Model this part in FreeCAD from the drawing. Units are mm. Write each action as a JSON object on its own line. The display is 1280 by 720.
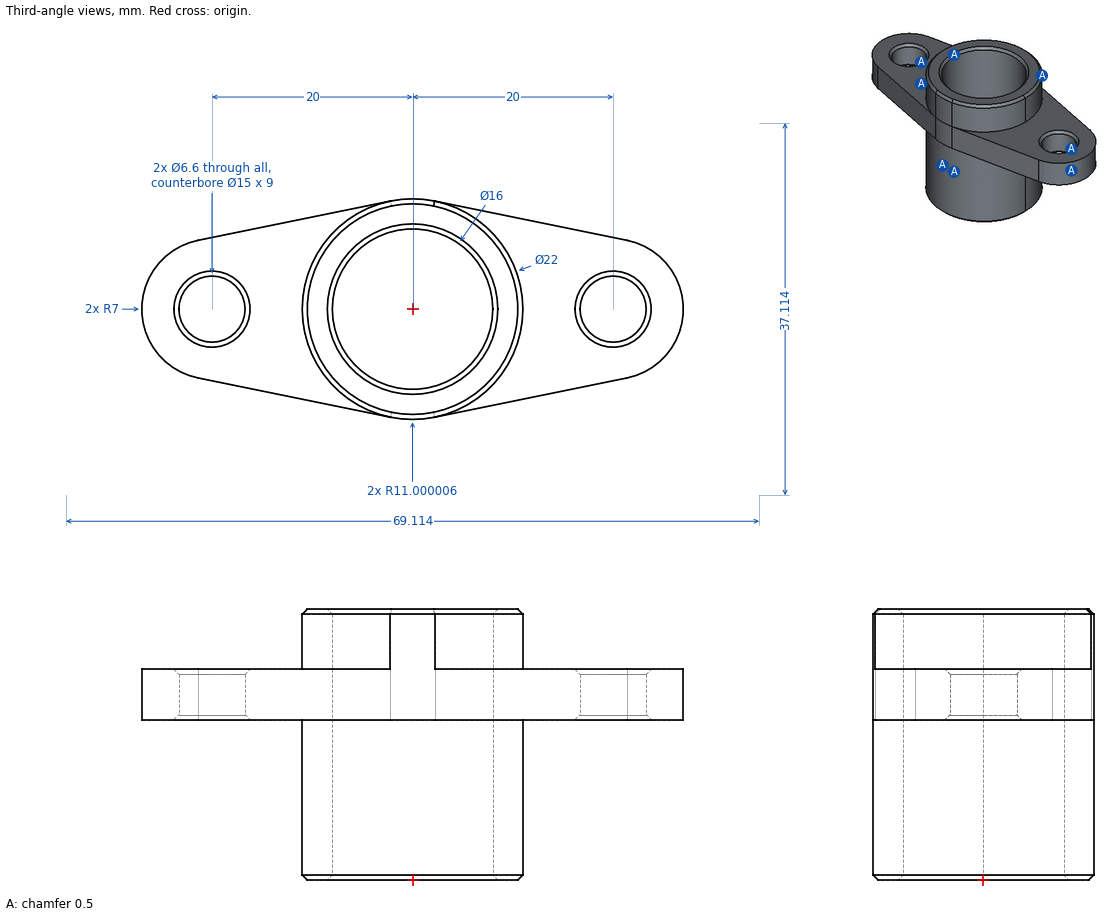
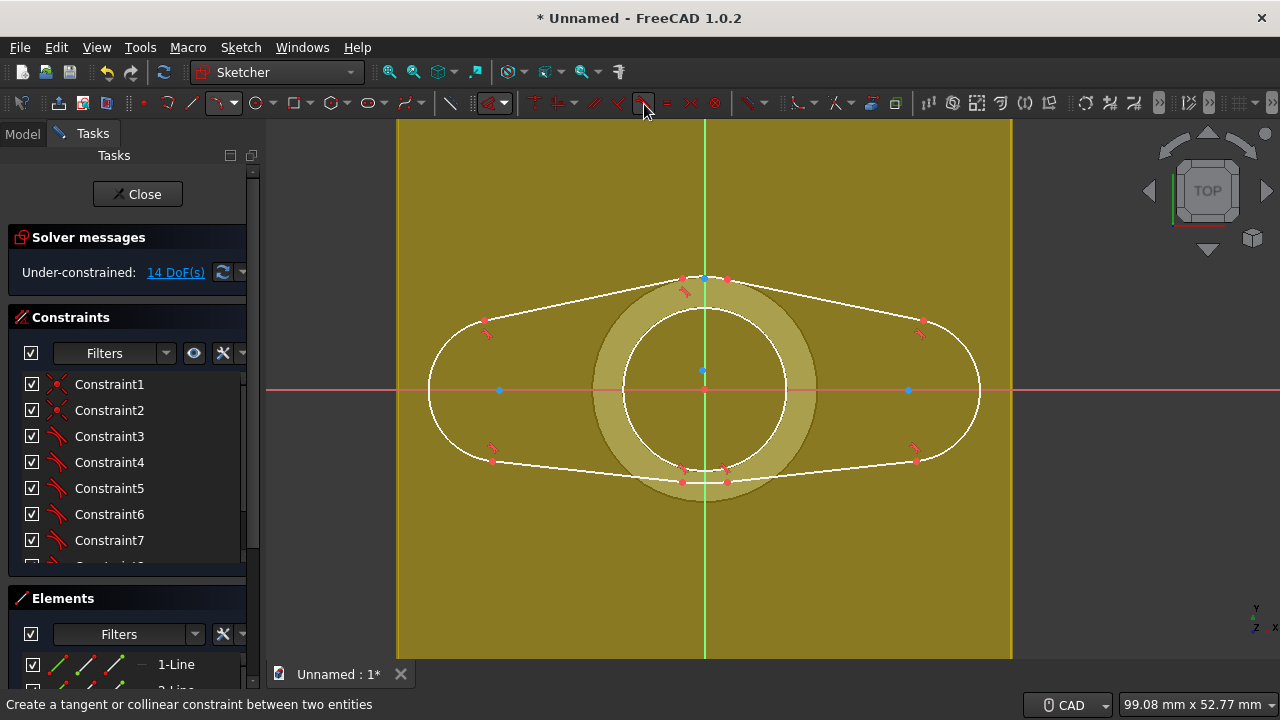
{"action": "left_click", "coordinate": [864, 308]}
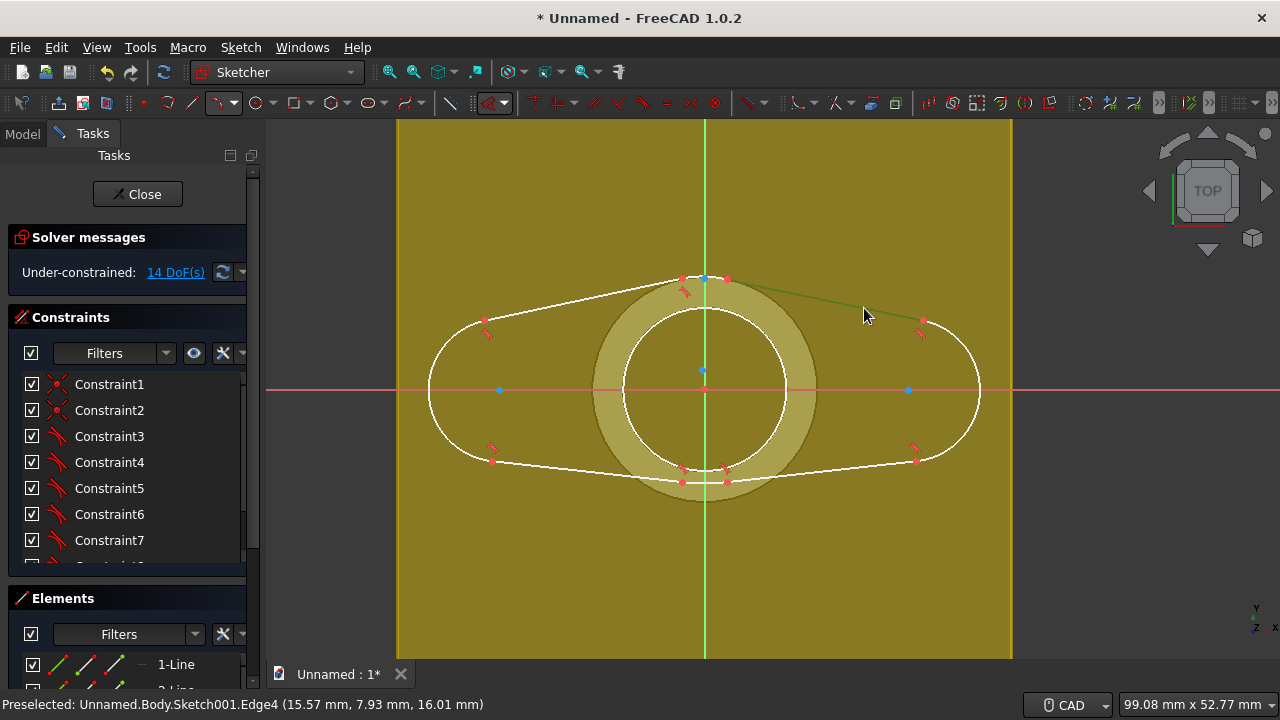
{"action": "scroll", "coordinate": [714, 277], "scroll_direction": "up", "scroll_amount": 3}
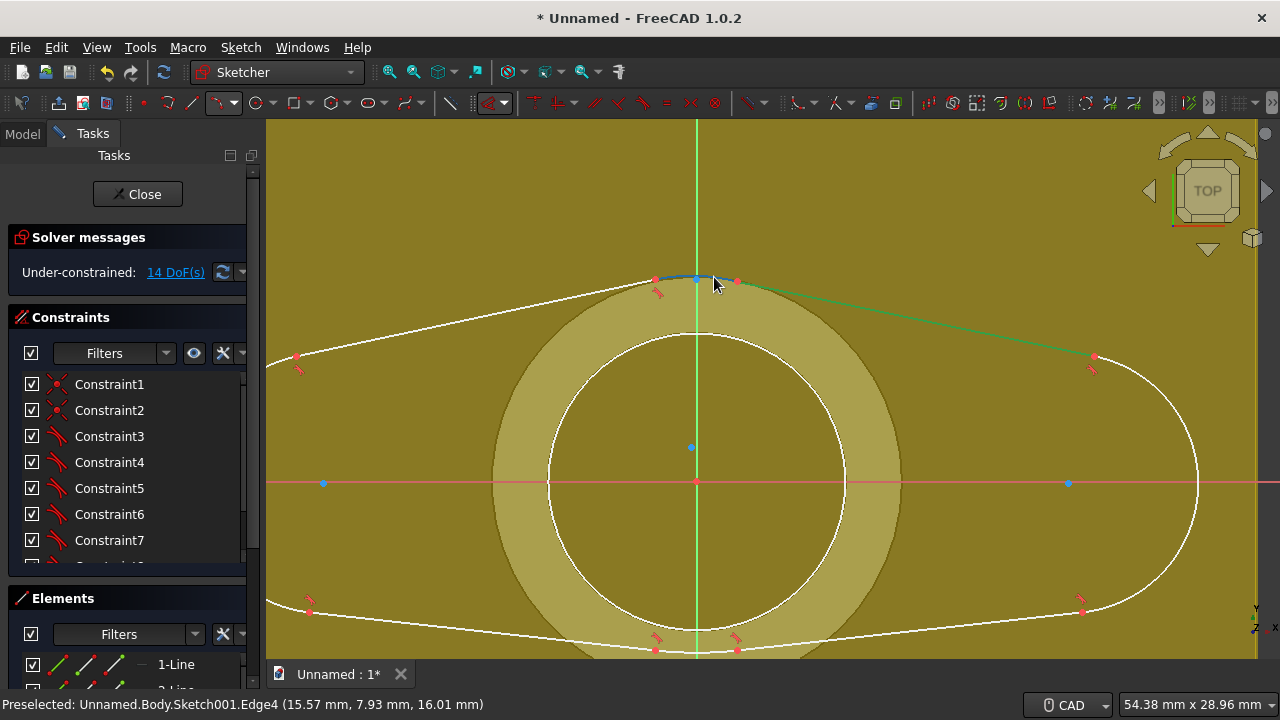
{"action": "left_click", "coordinate": [713, 277]}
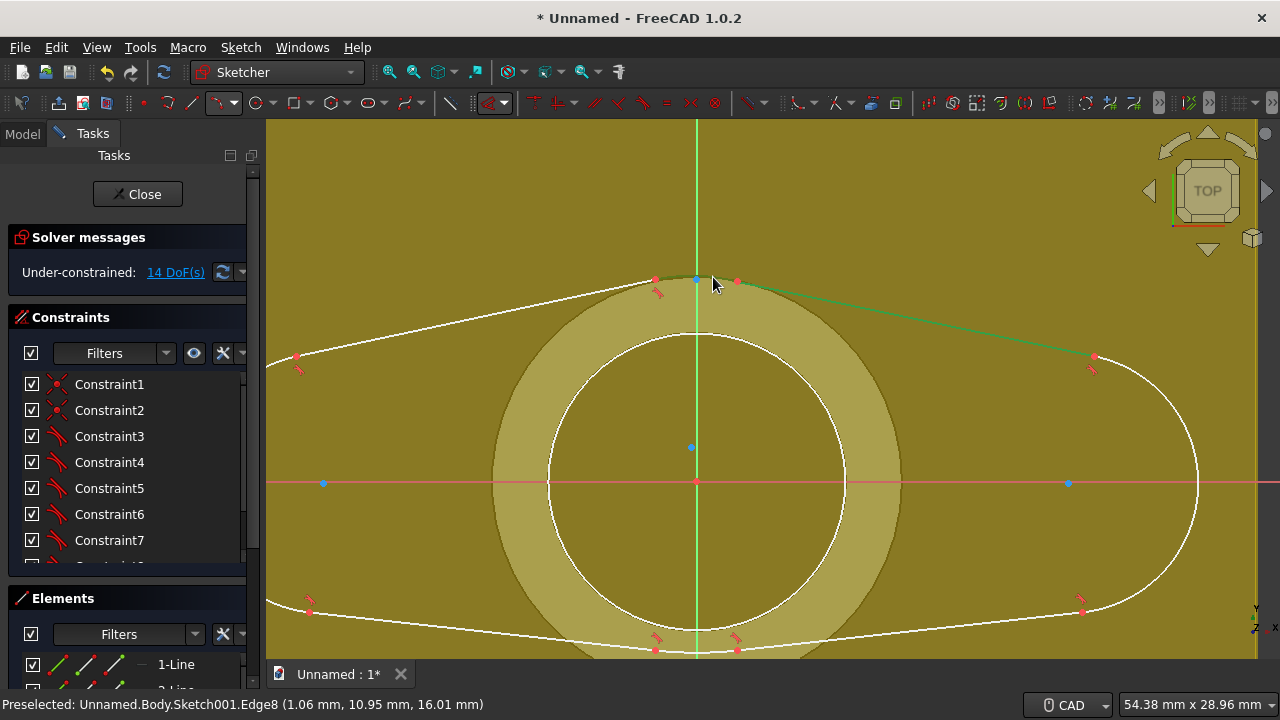
{"action": "key", "text": "t"}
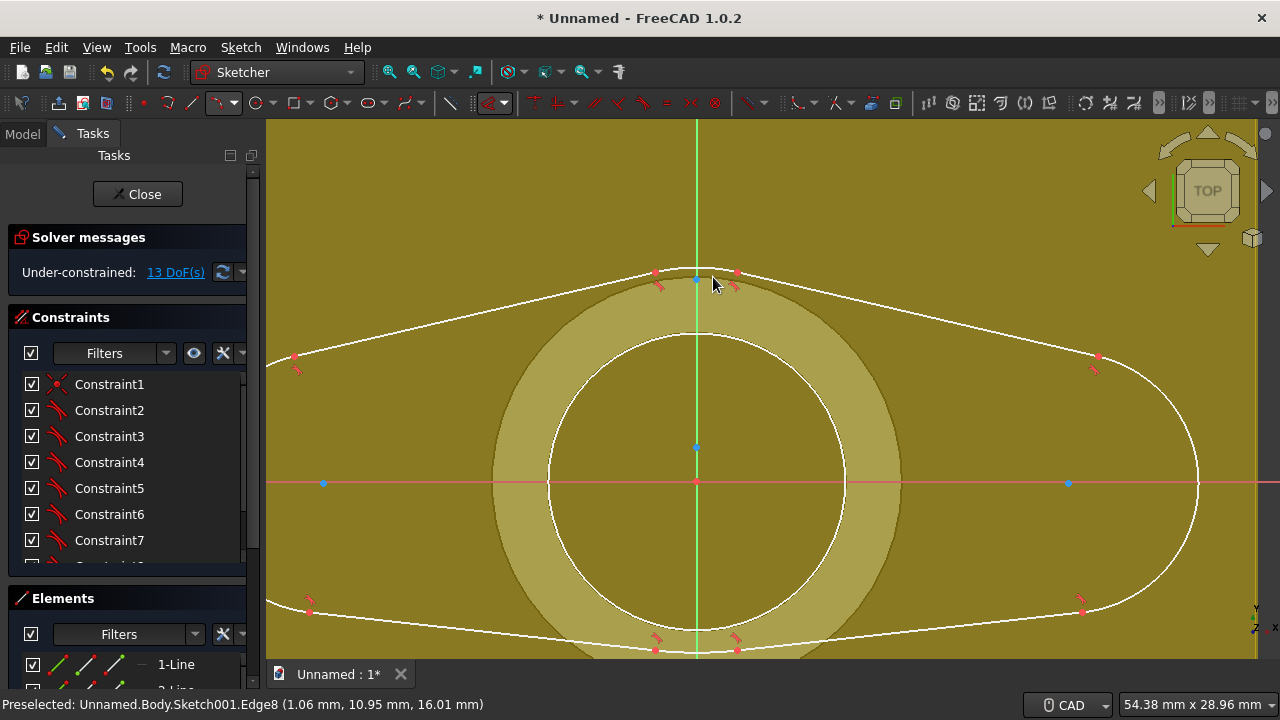
{"action": "left_click", "coordinate": [802, 376]}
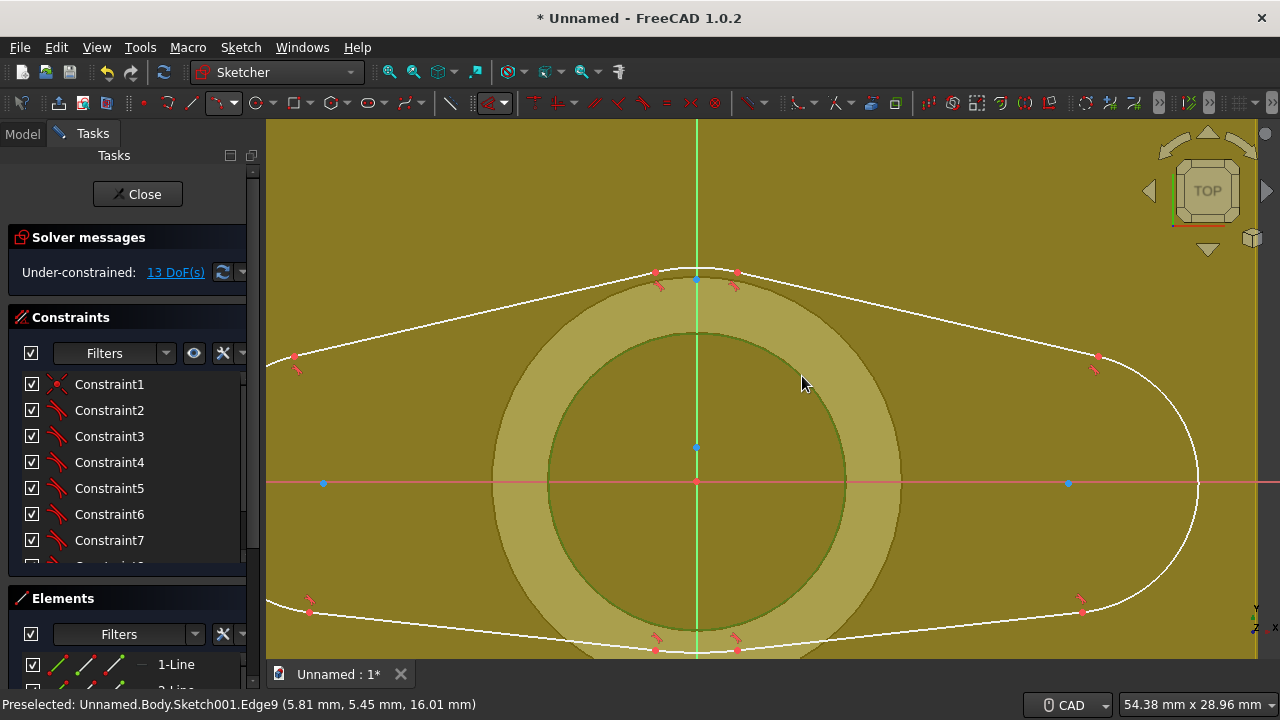
{"action": "scroll", "coordinate": [714, 276], "scroll_direction": "down", "scroll_amount": 3}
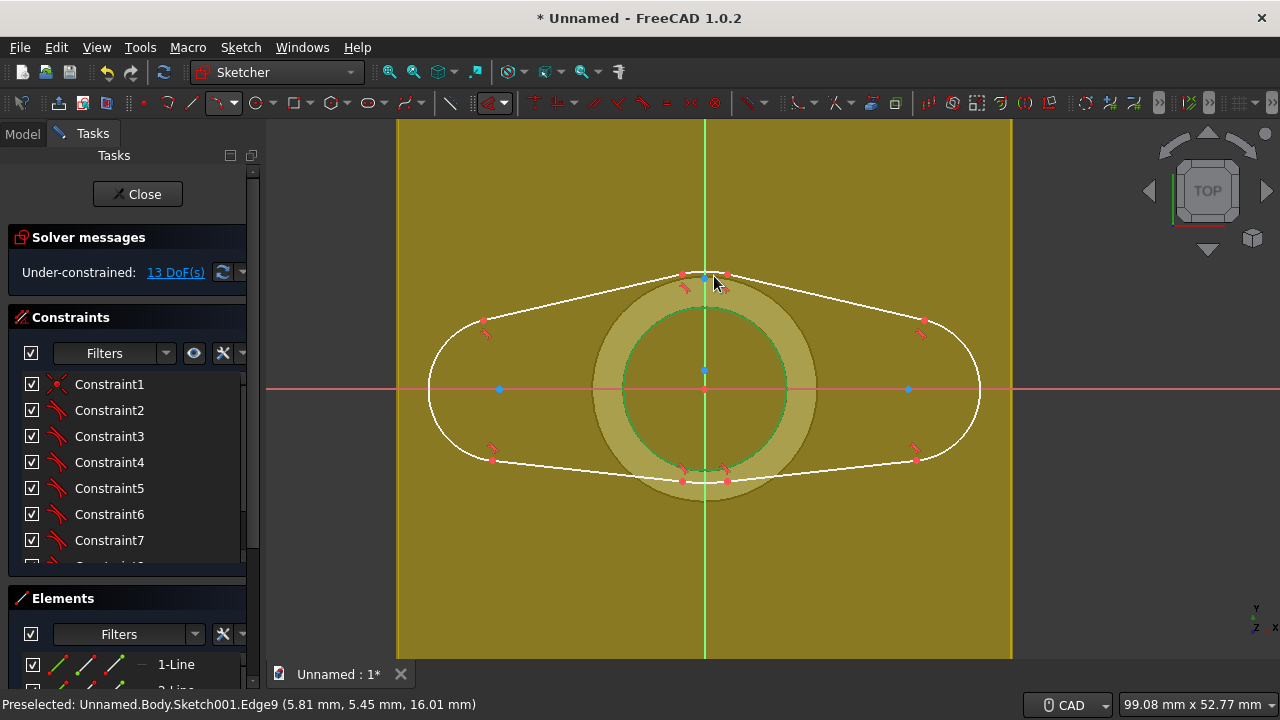
{"action": "scroll", "coordinate": [696, 483], "scroll_direction": "up", "scroll_amount": 3}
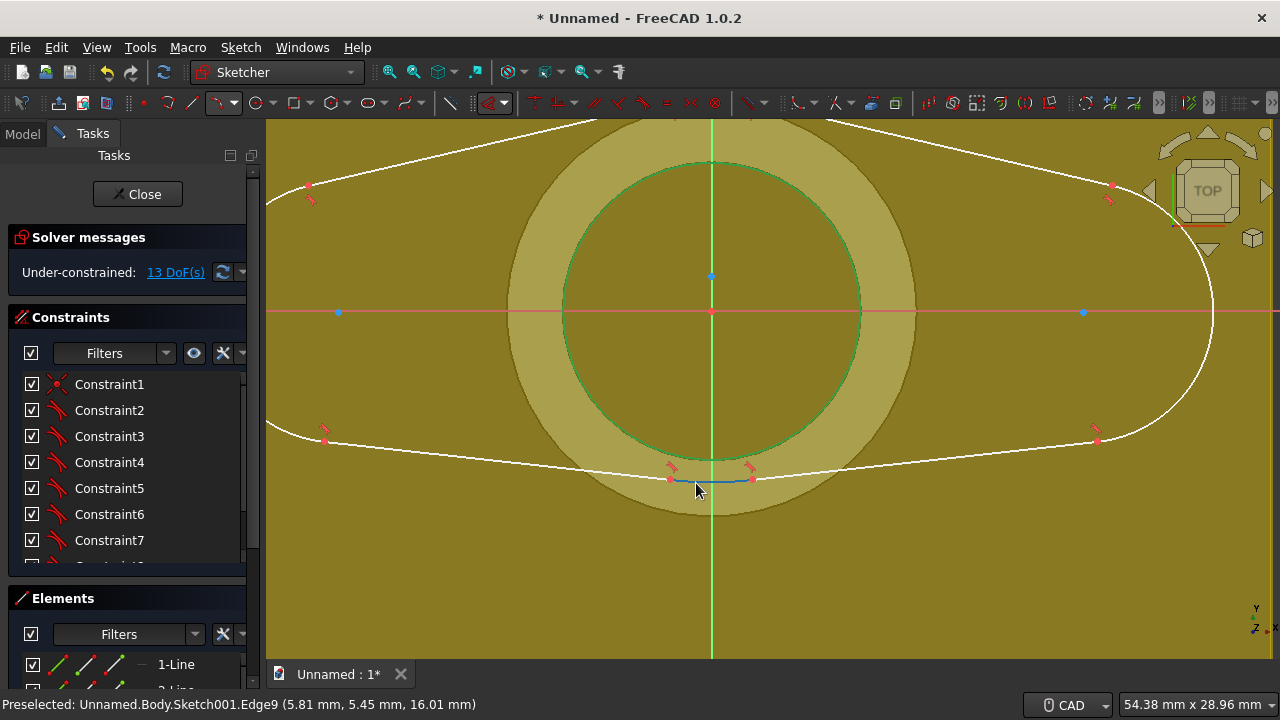
{"action": "left_click", "coordinate": [695, 482]}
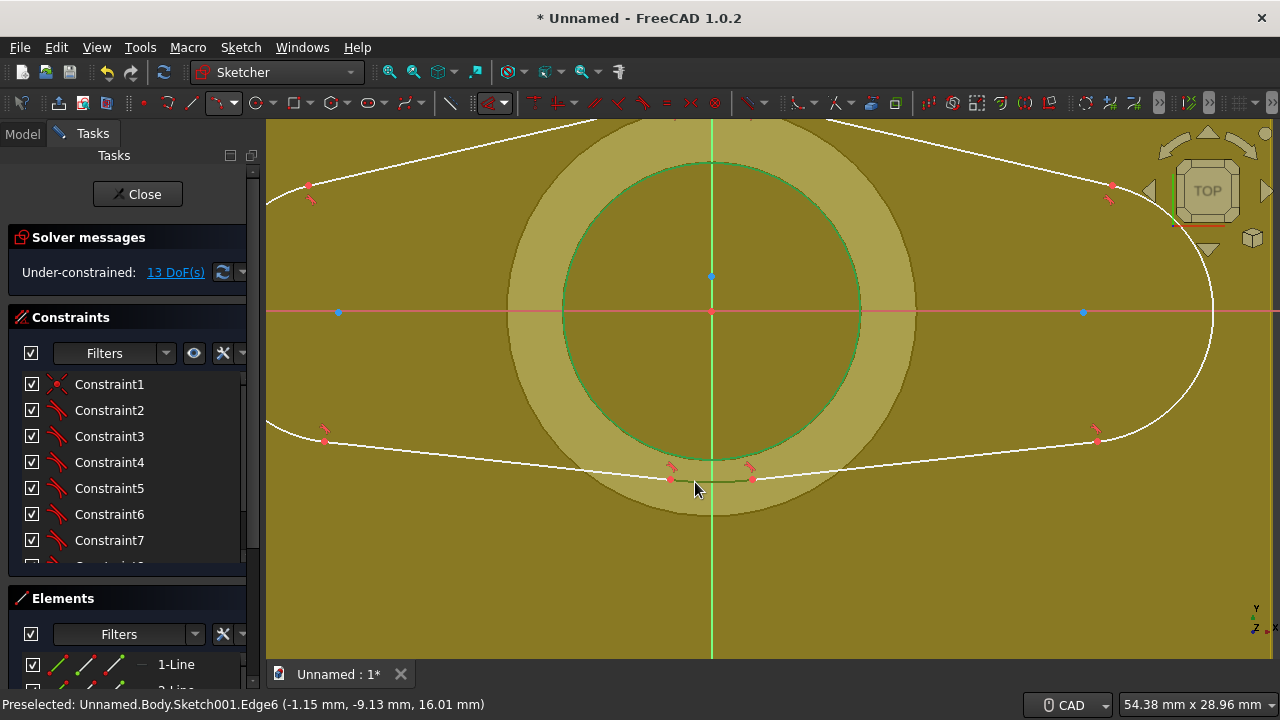
{"action": "left_click", "coordinate": [534, 104]}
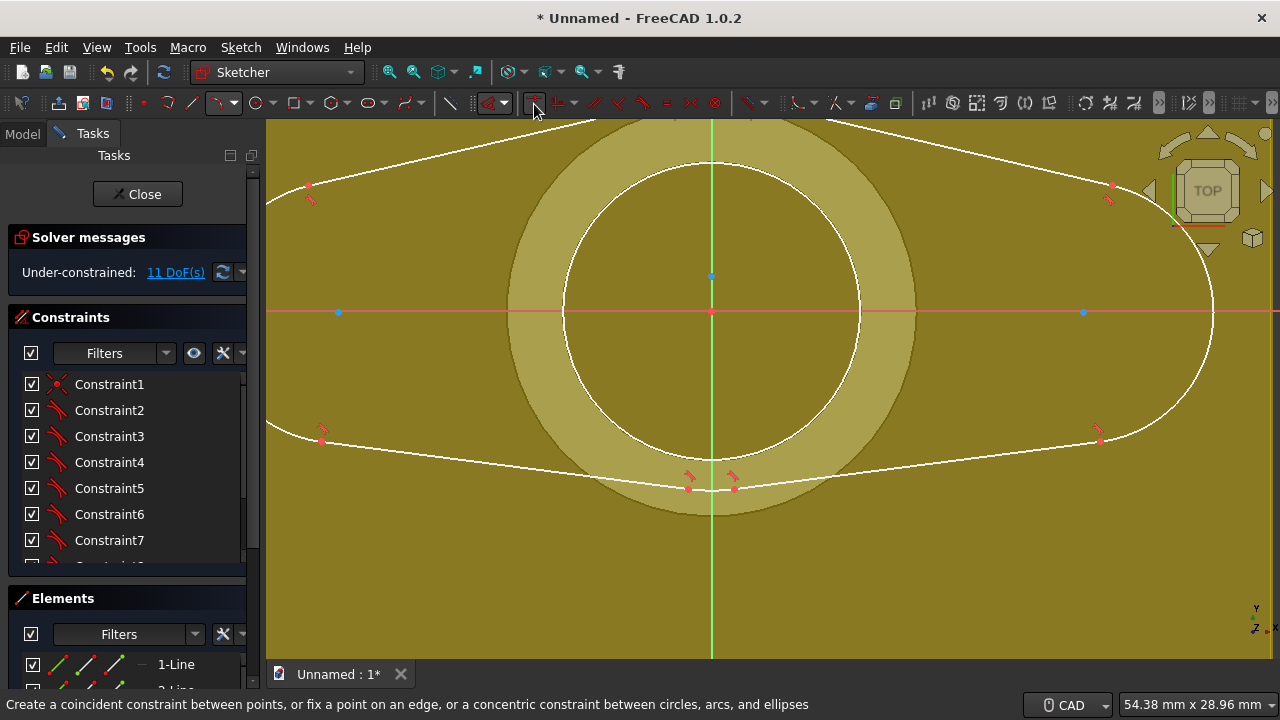
{"action": "left_click", "coordinate": [816, 206]}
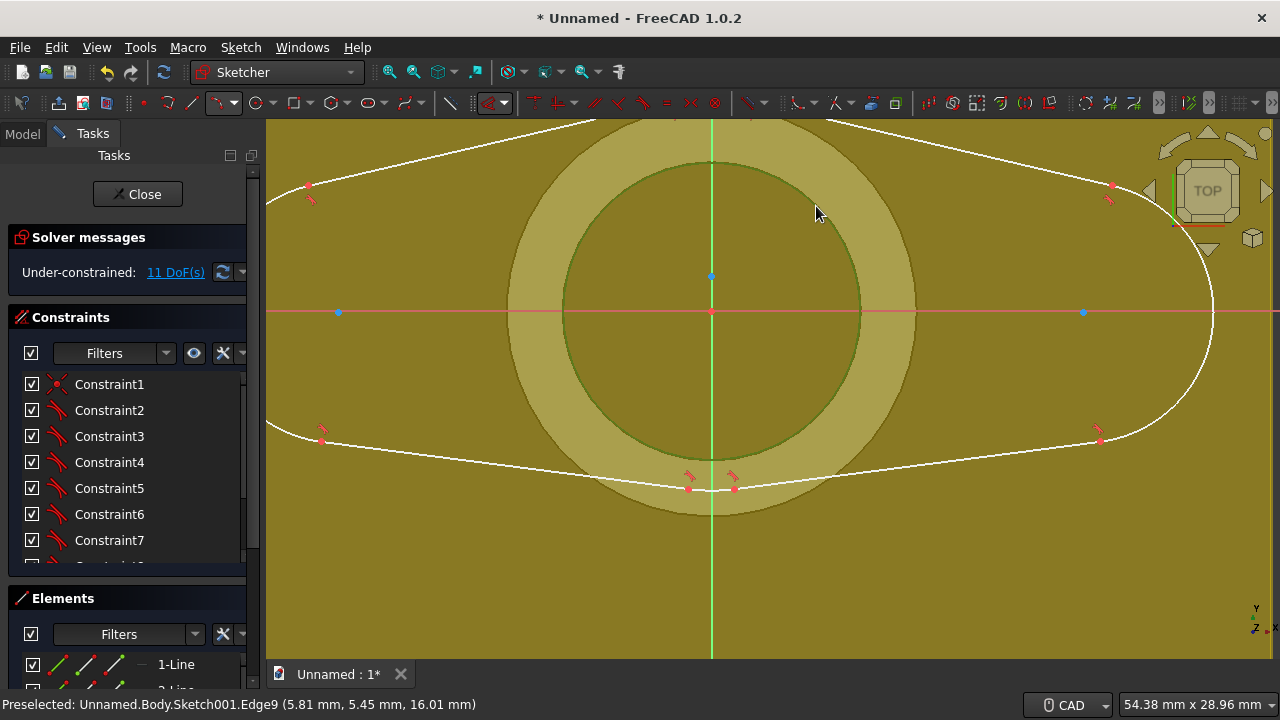
{"action": "scroll", "coordinate": [696, 483], "scroll_direction": "down", "scroll_amount": 3}